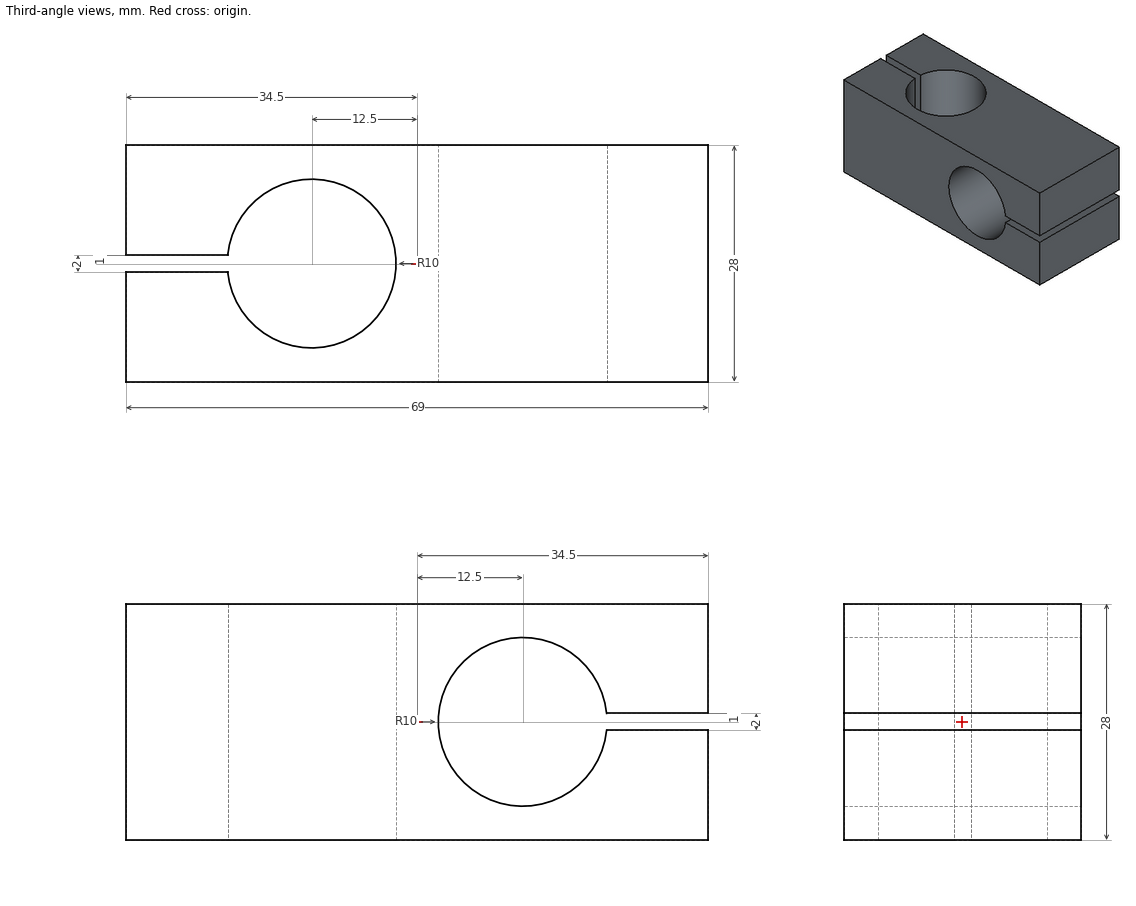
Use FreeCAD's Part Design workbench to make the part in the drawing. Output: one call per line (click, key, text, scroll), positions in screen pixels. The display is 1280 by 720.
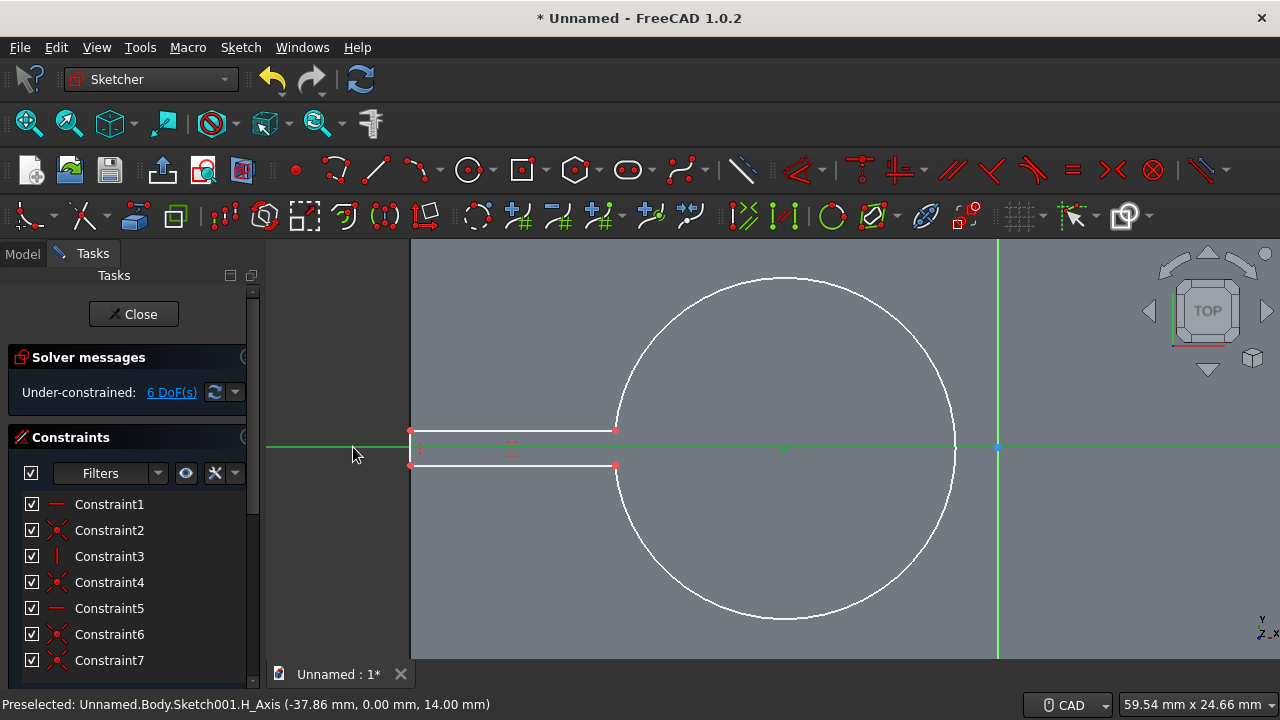
click(860, 170)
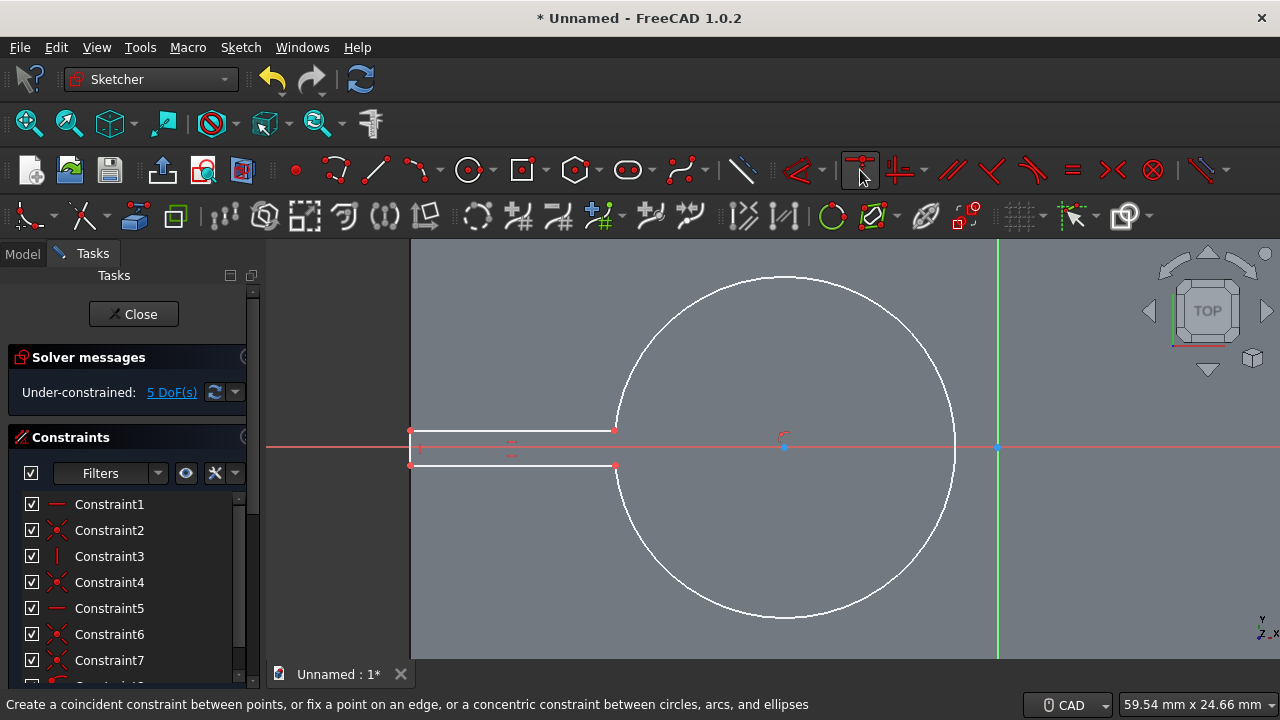
key(d)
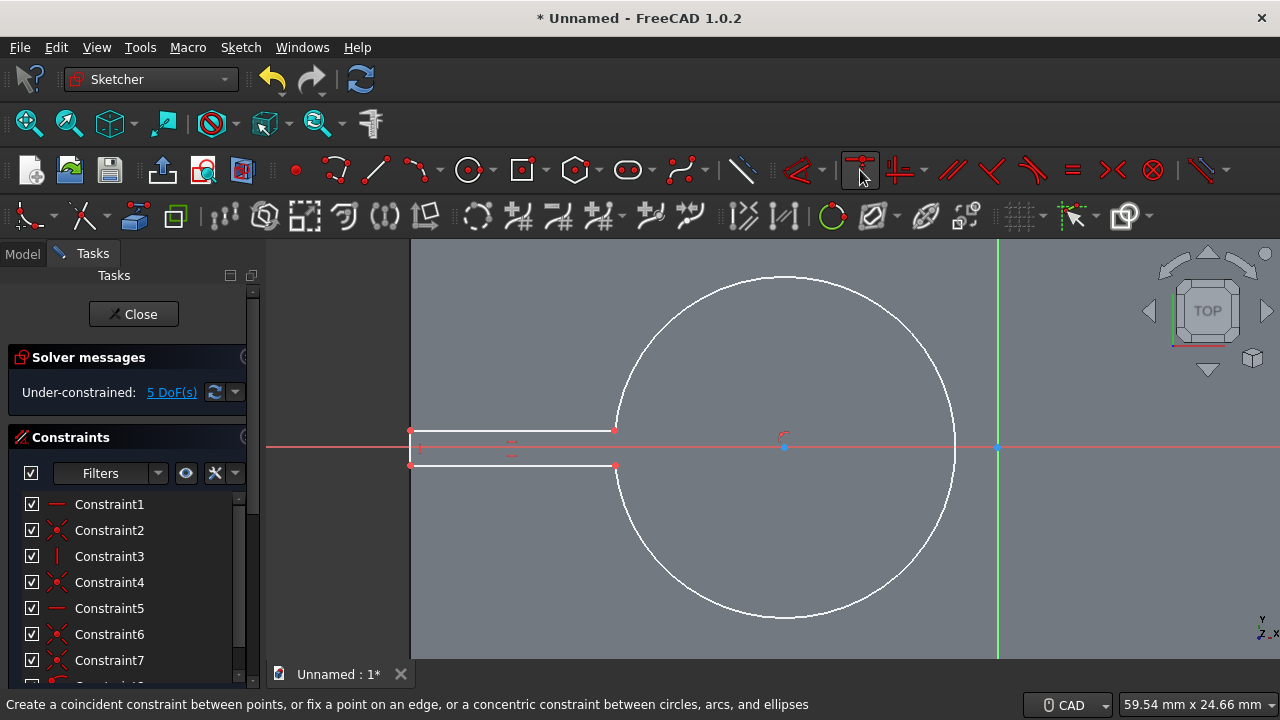
click(845, 607)
click(938, 579)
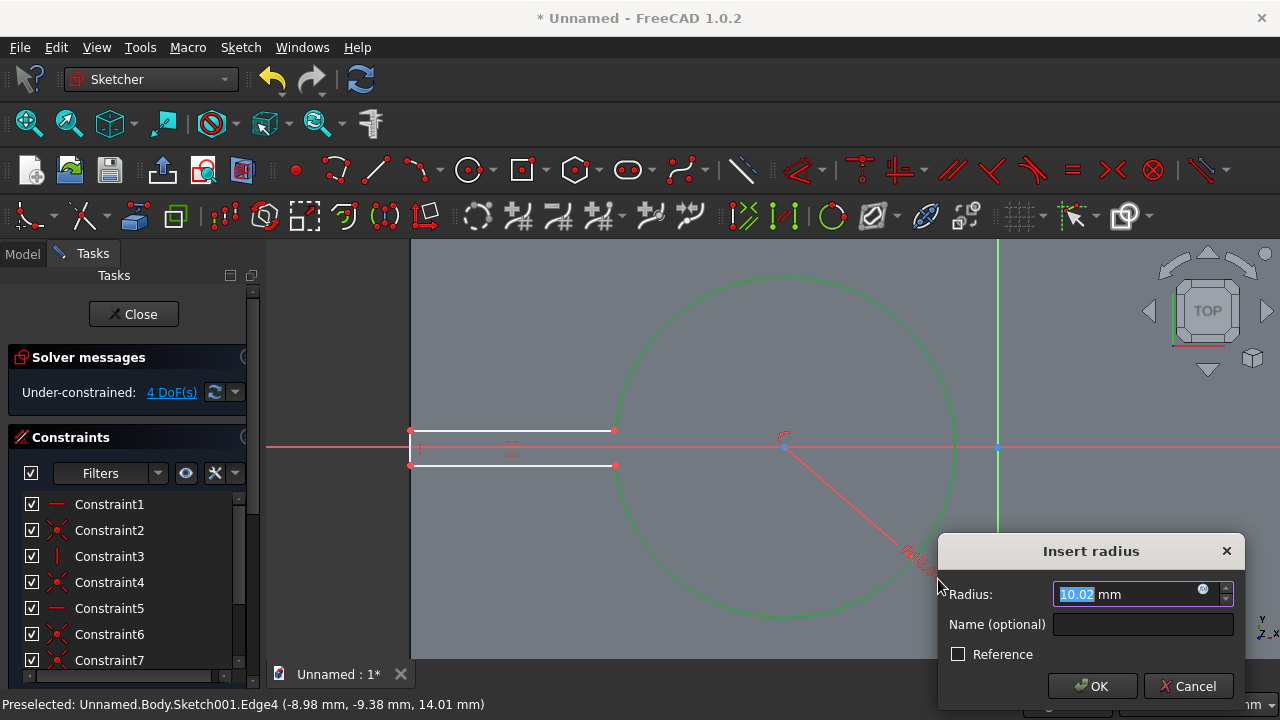
text(10)
key(Return)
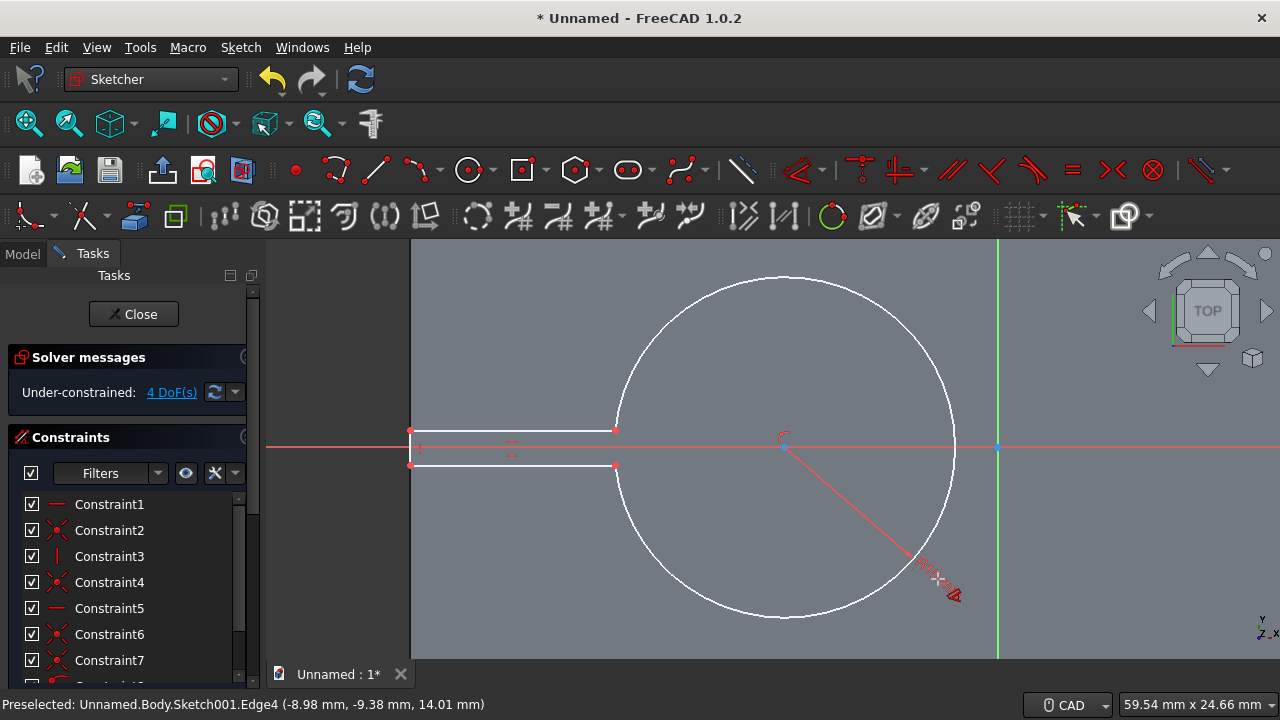
click(410, 445)
click(376, 461)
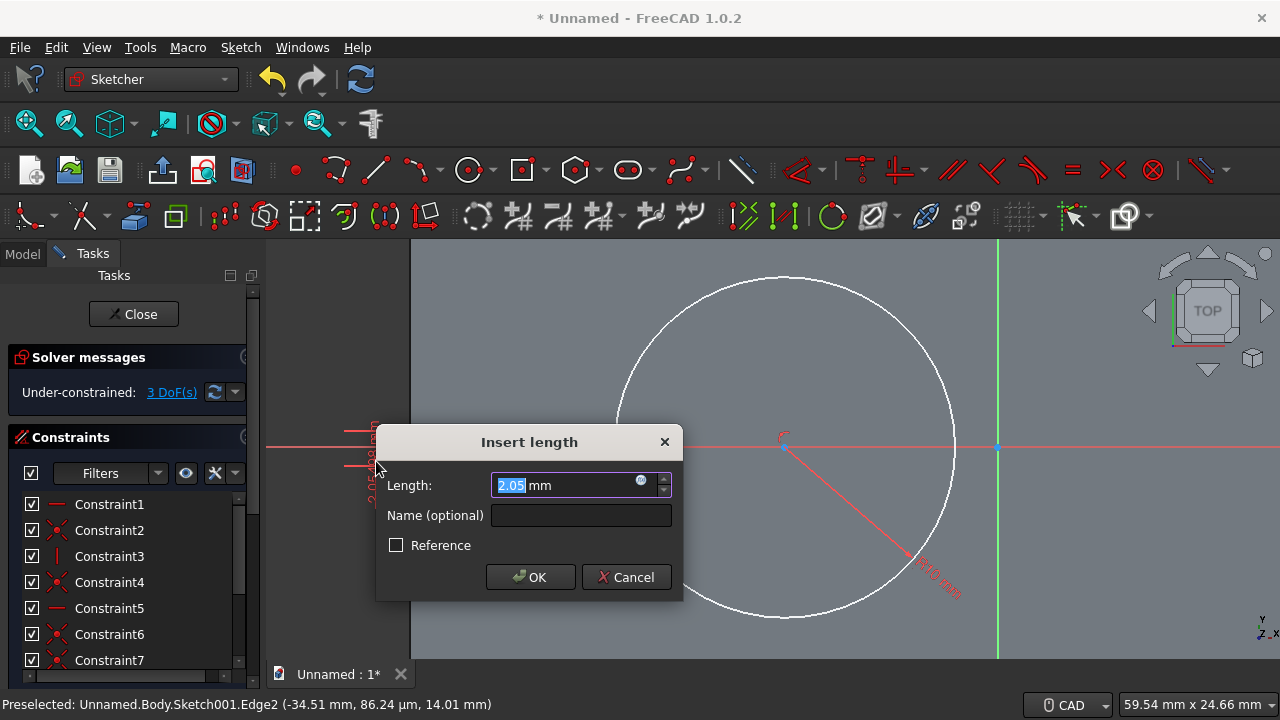
text(2)
key(Return)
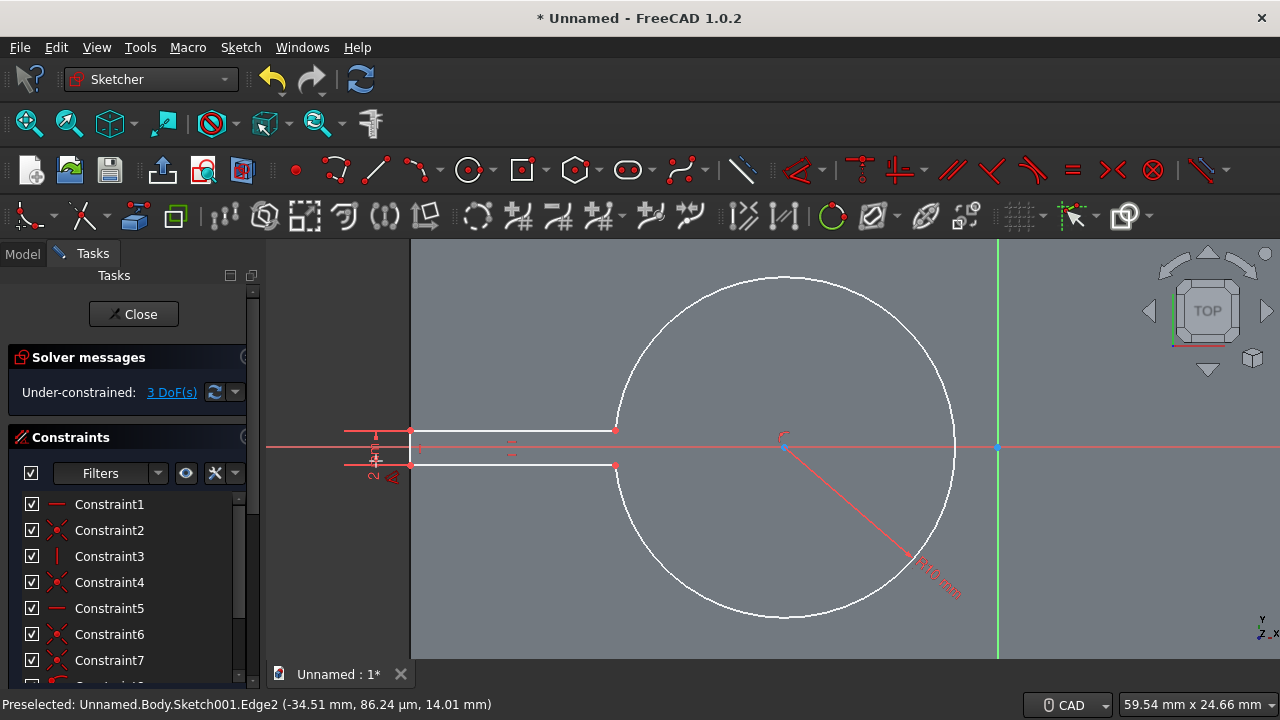
scroll(615, 431, up, 5)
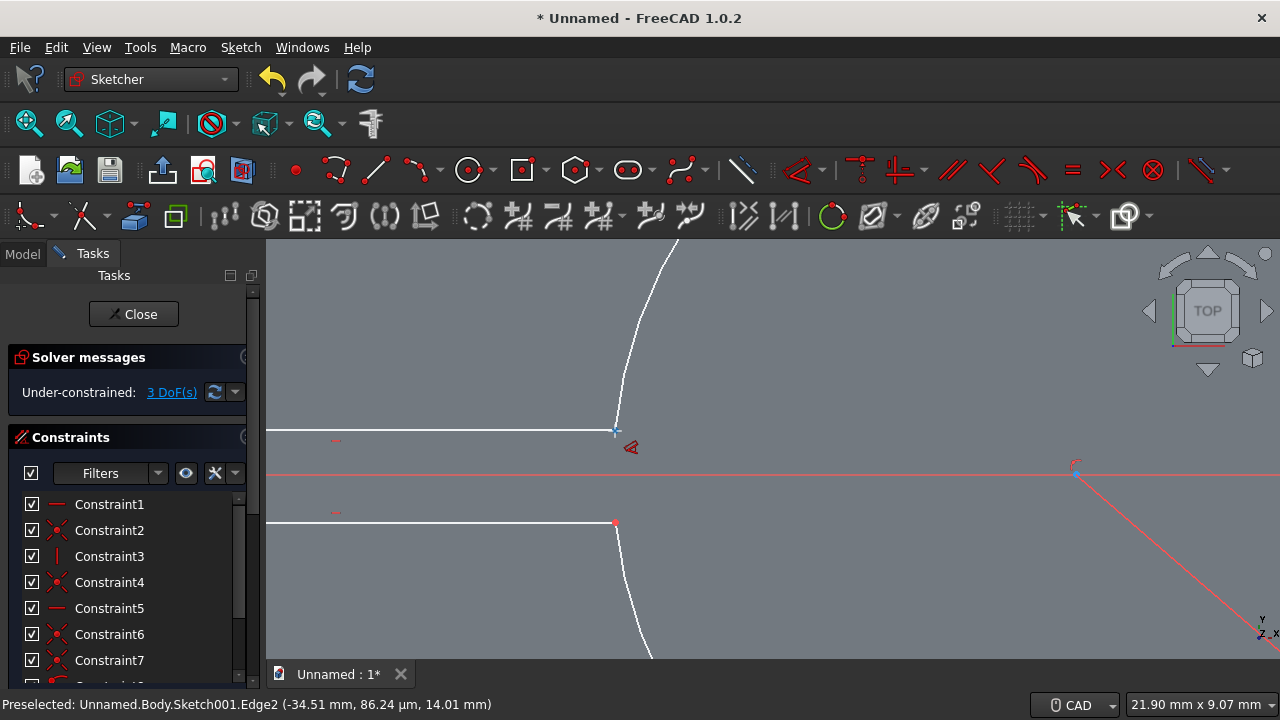
click(615, 430)
click(581, 453)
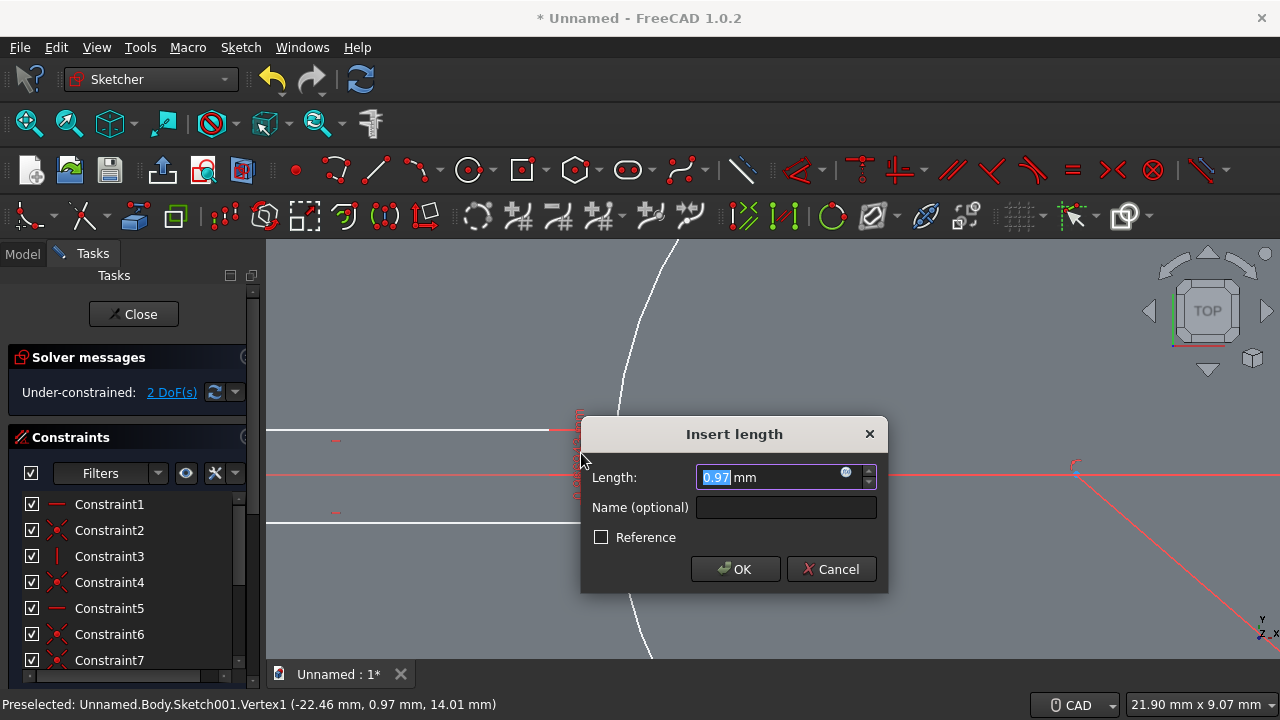
text(1)
key(Return)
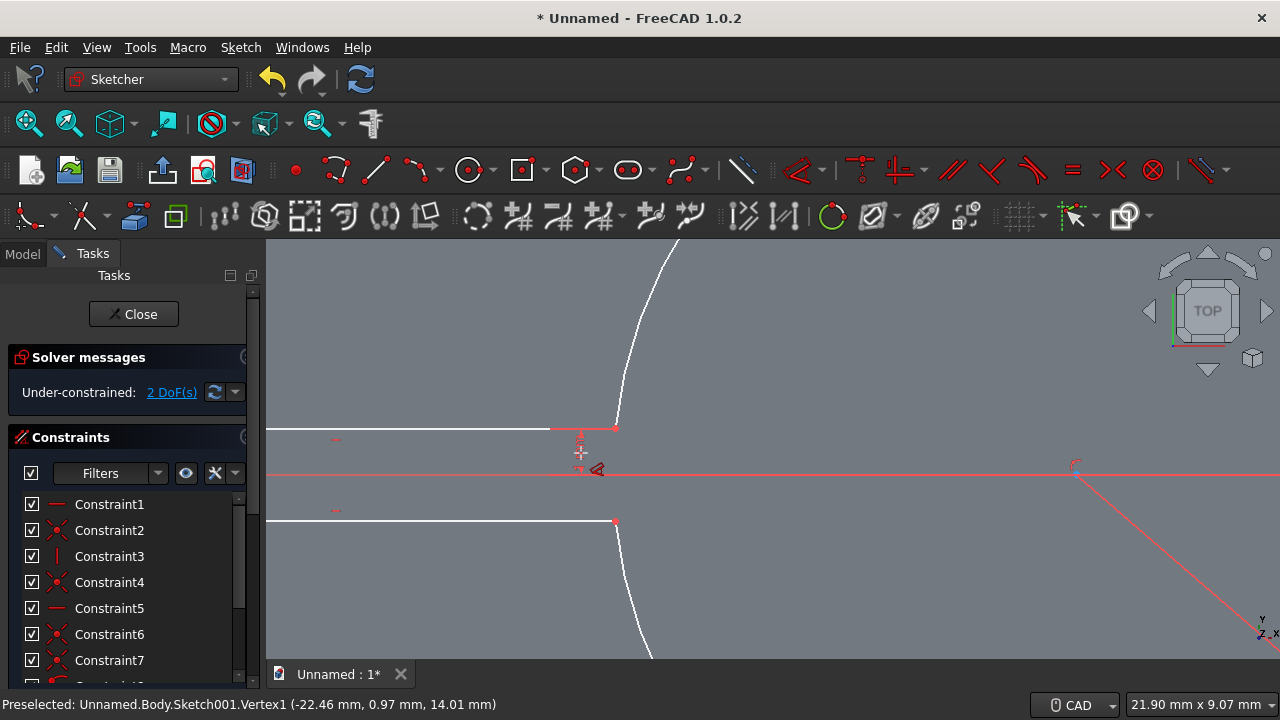
scroll(616, 434, down, 5)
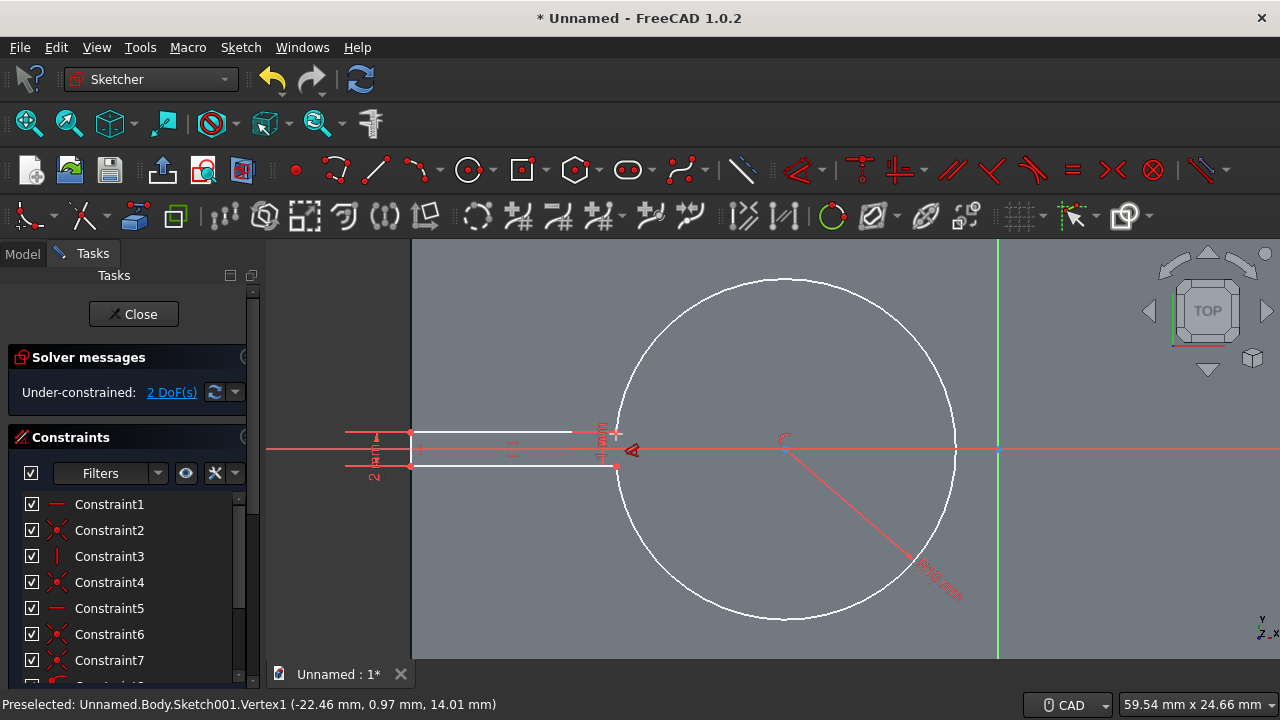
click(411, 432)
click(705, 398)